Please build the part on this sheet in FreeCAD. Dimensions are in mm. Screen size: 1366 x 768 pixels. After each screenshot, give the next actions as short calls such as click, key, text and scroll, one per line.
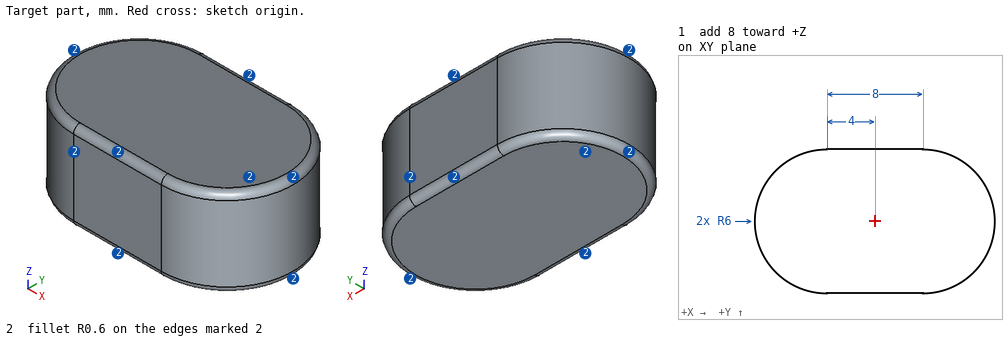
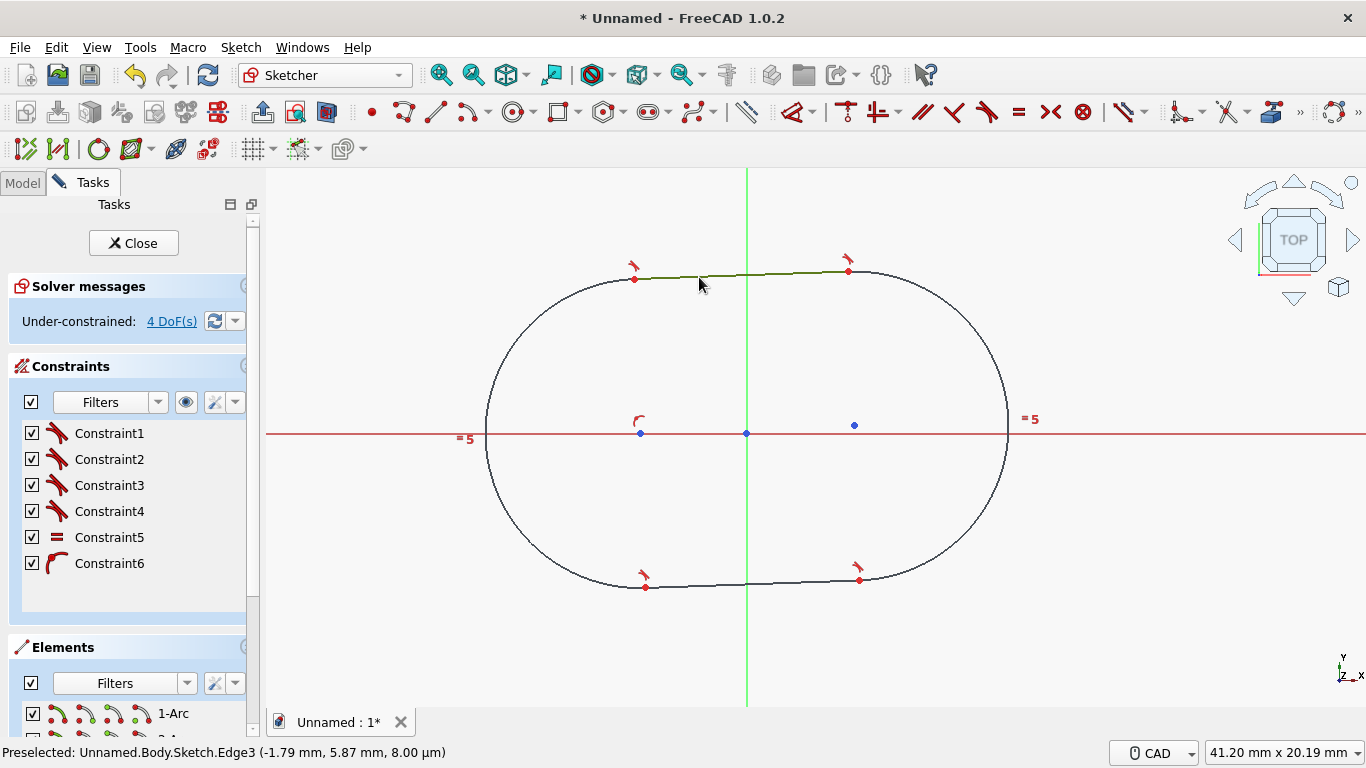
key(h)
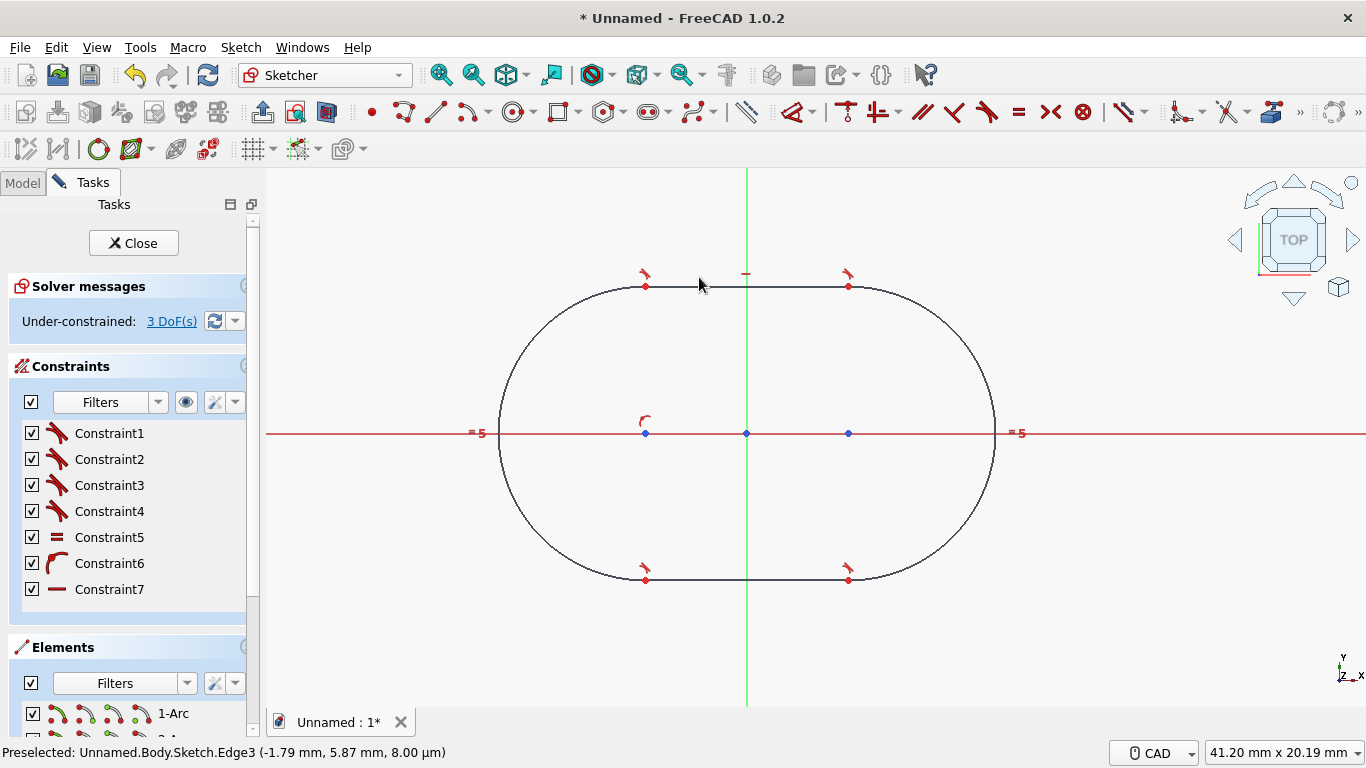
click(527, 347)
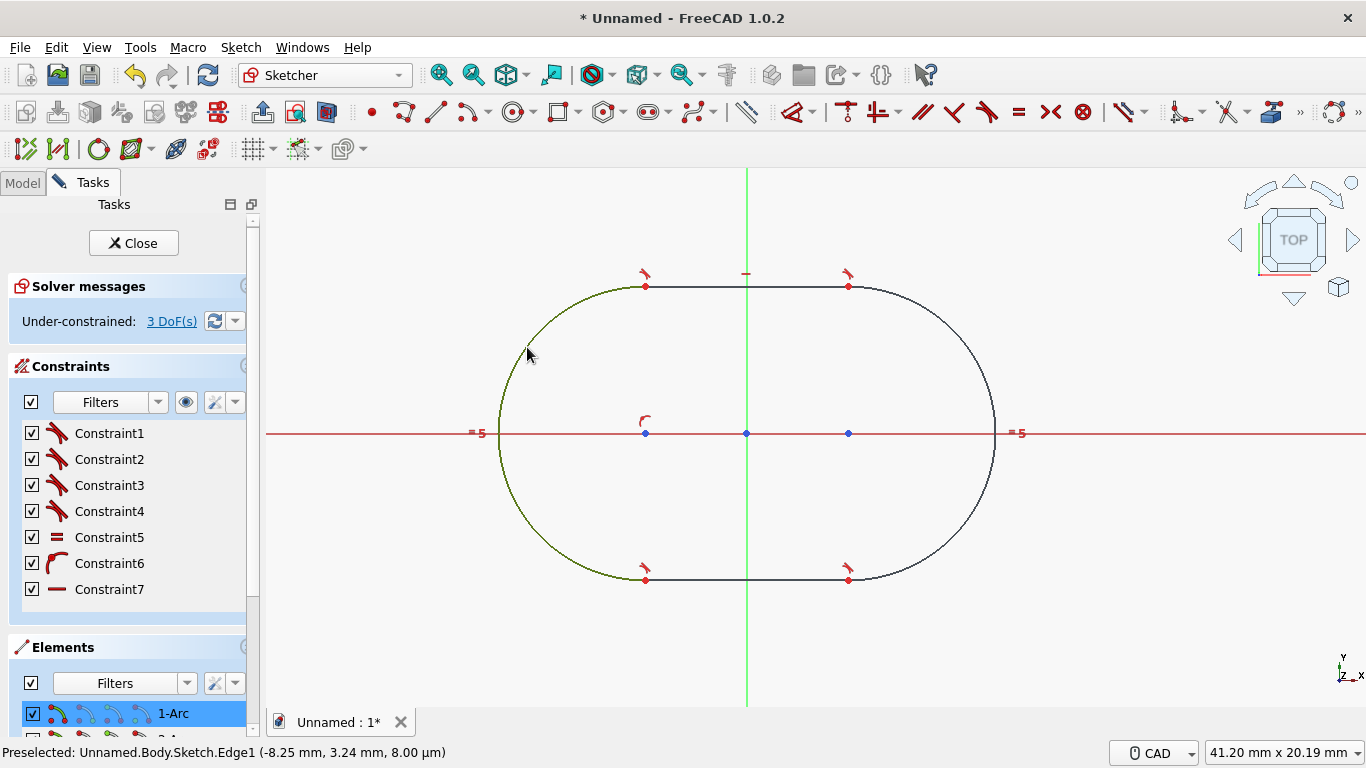
key(k)
key(r)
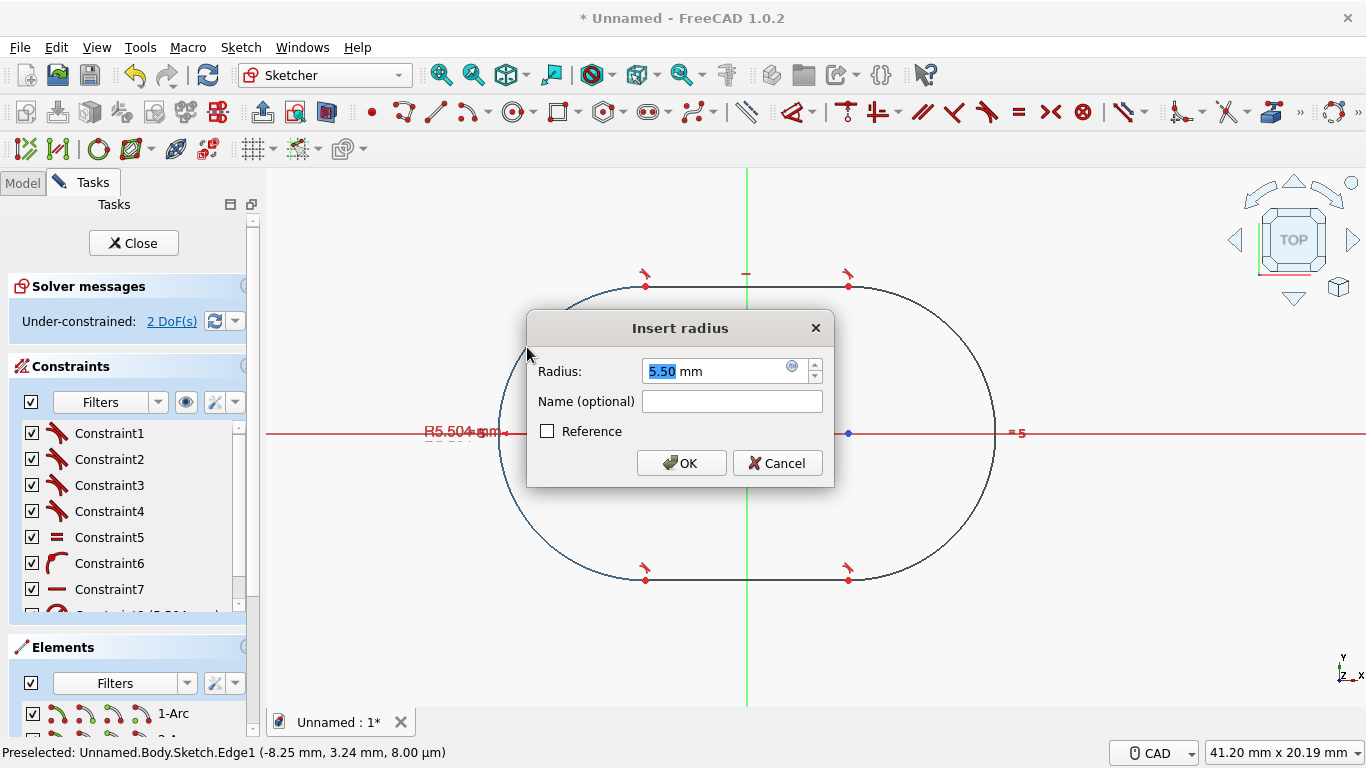
text(6)
key(Return)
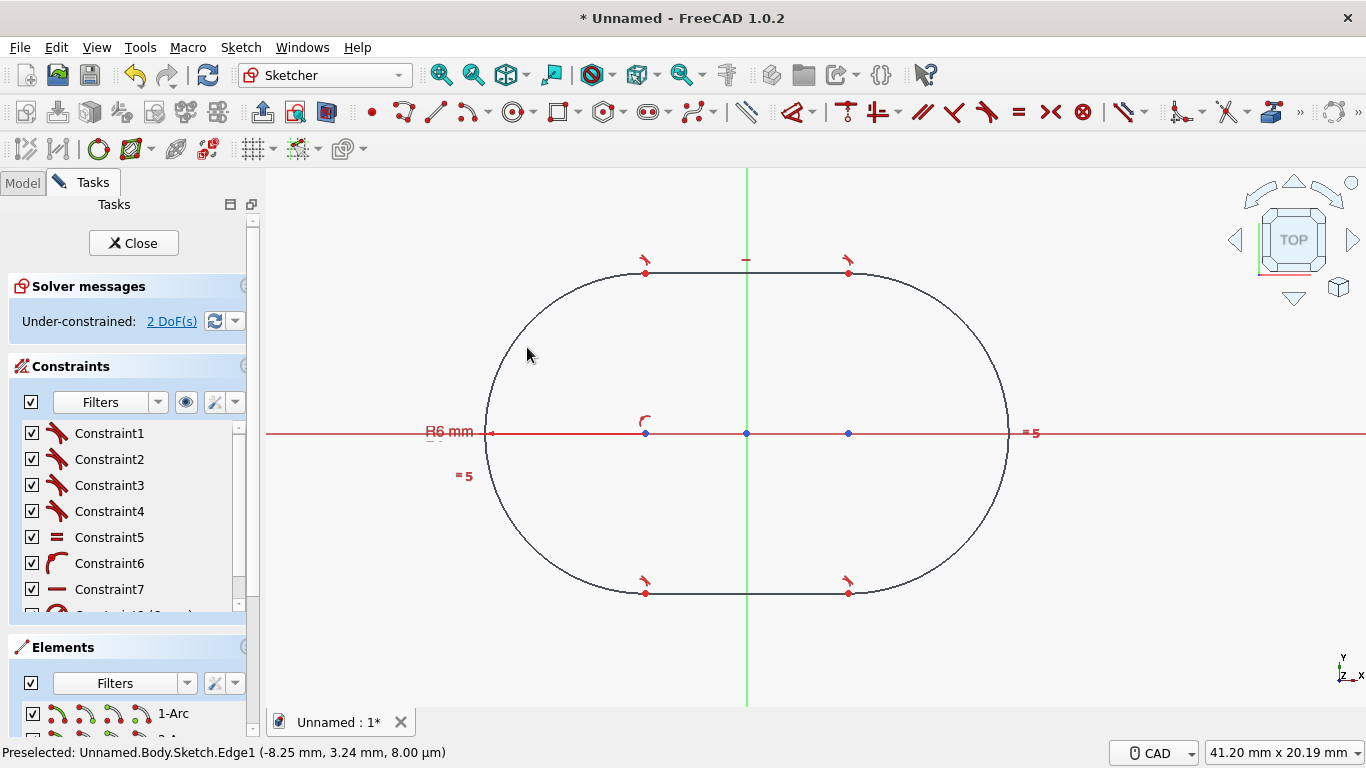
click(706, 273)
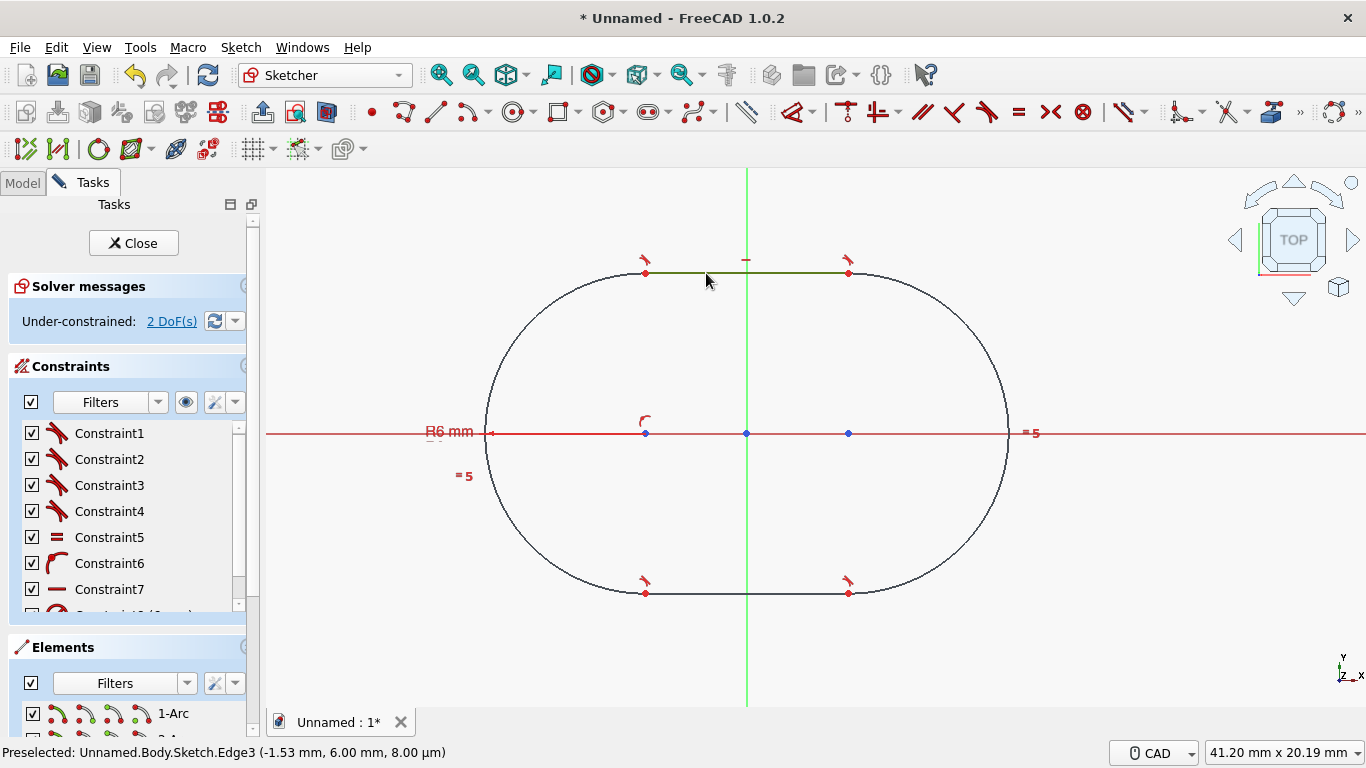
key(l)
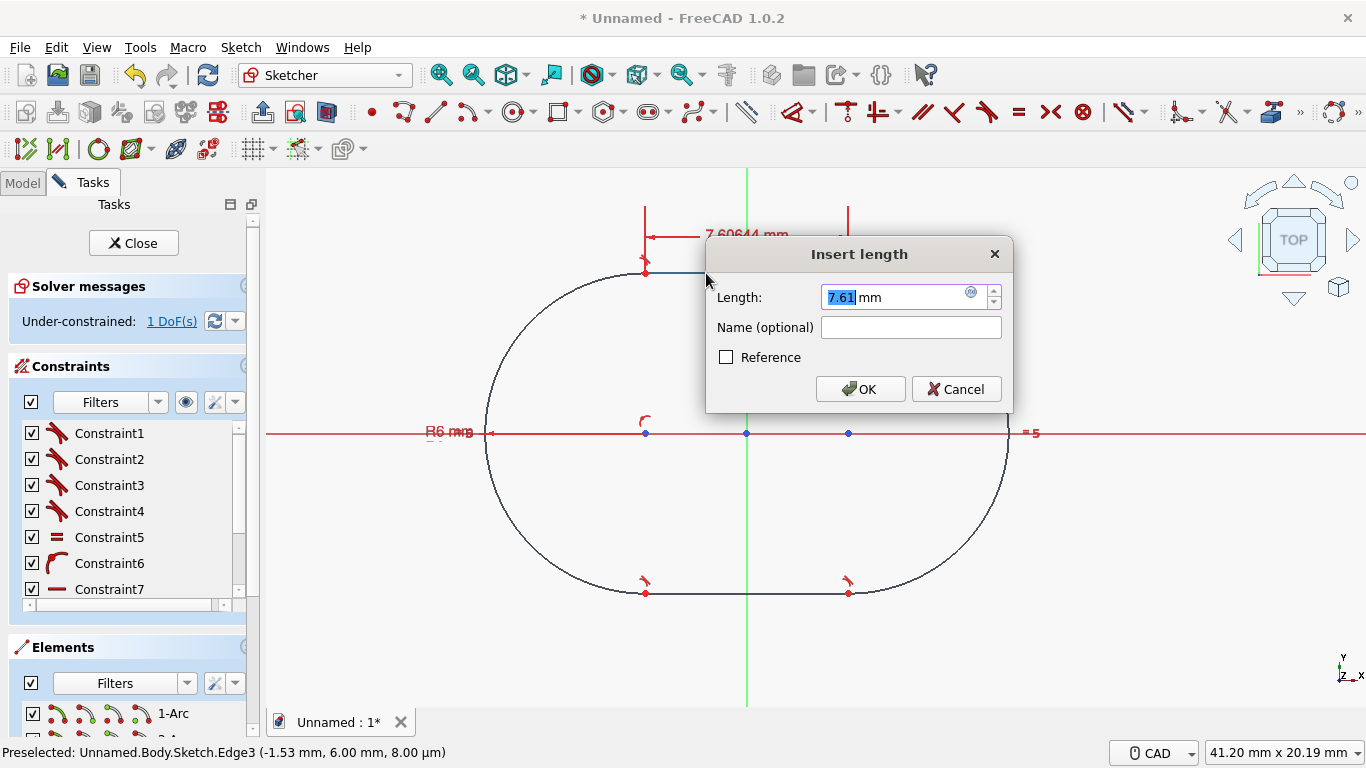
text(8)
key(Return)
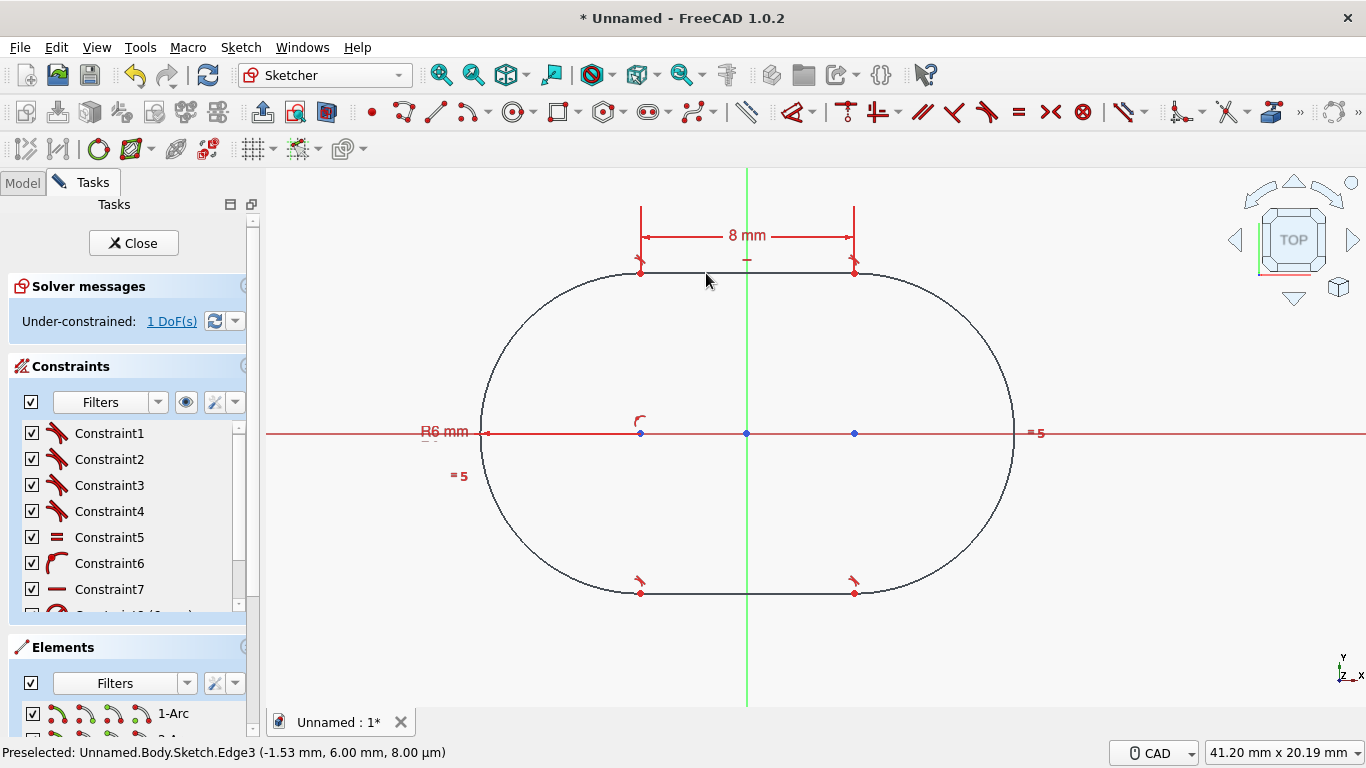
click(641, 273)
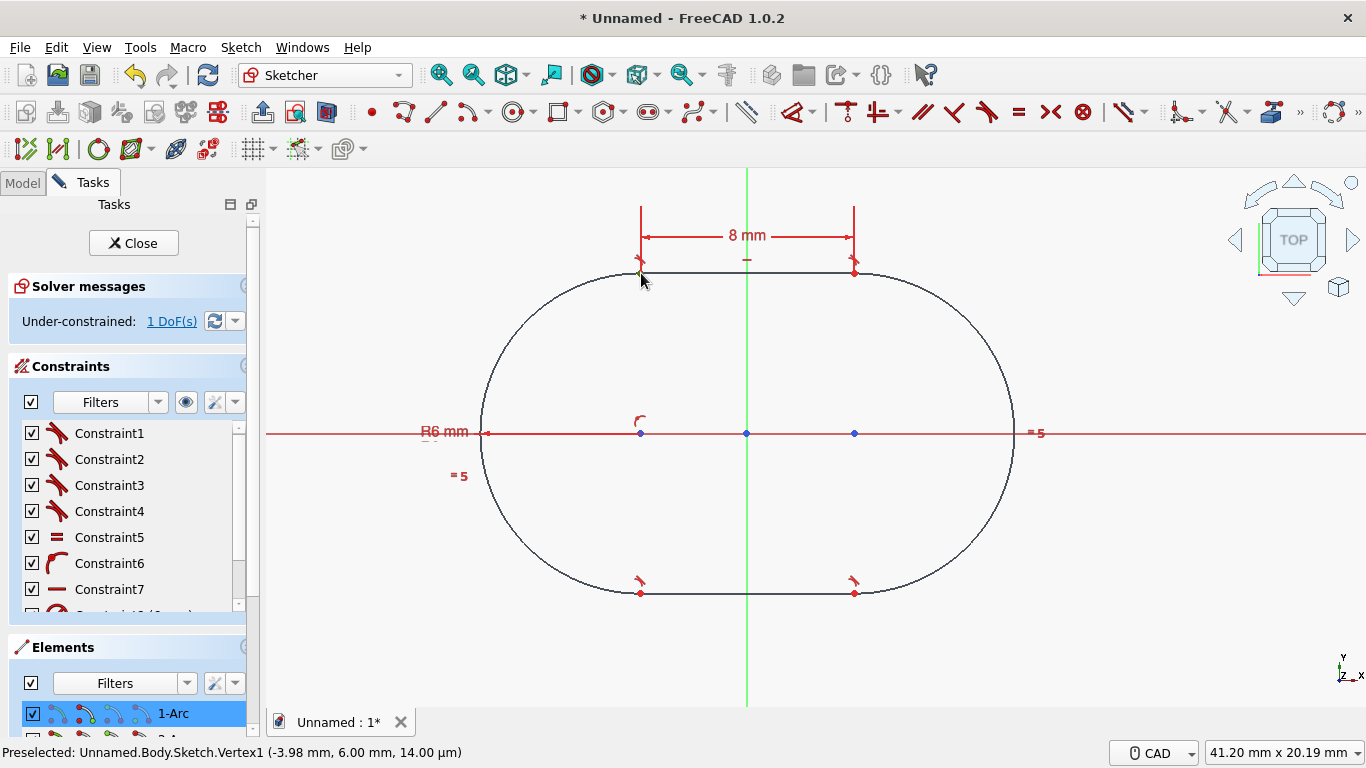
key(l)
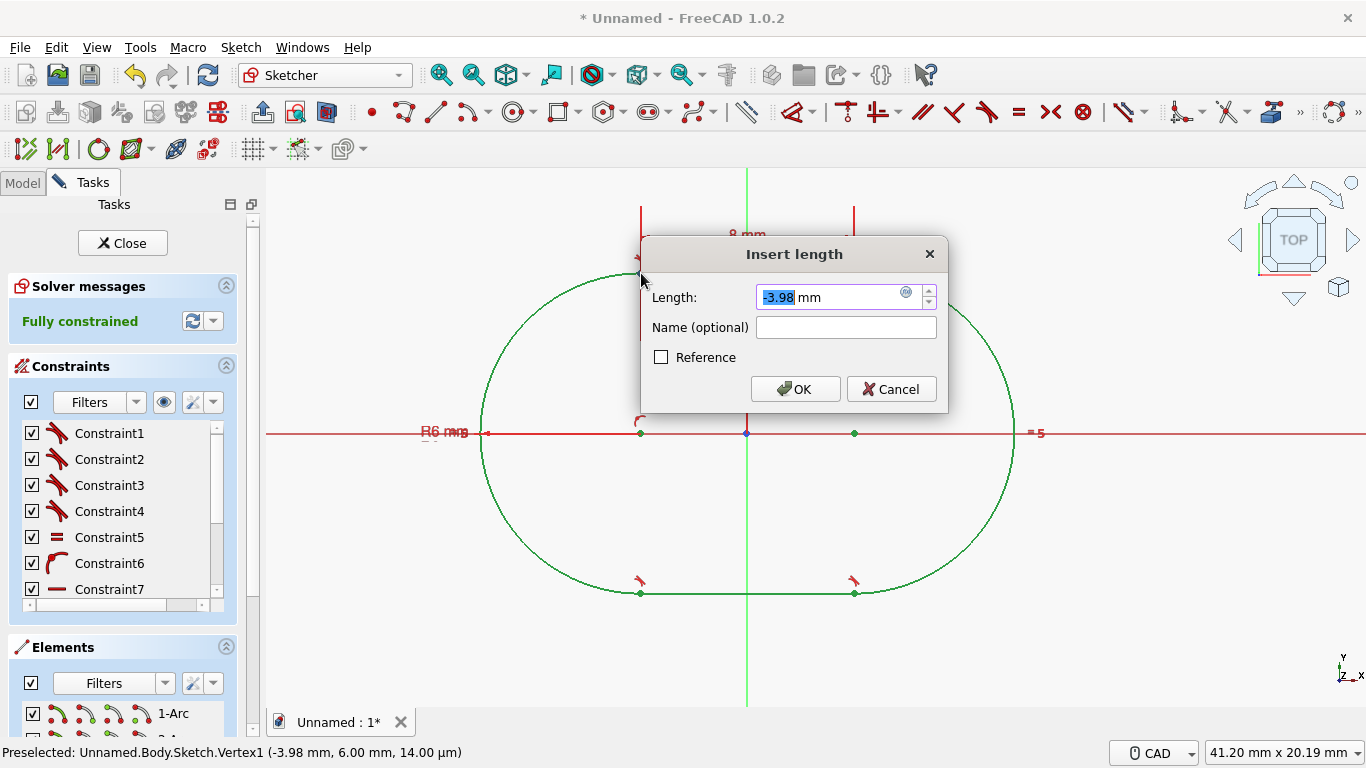
text(-4)
key(Return)